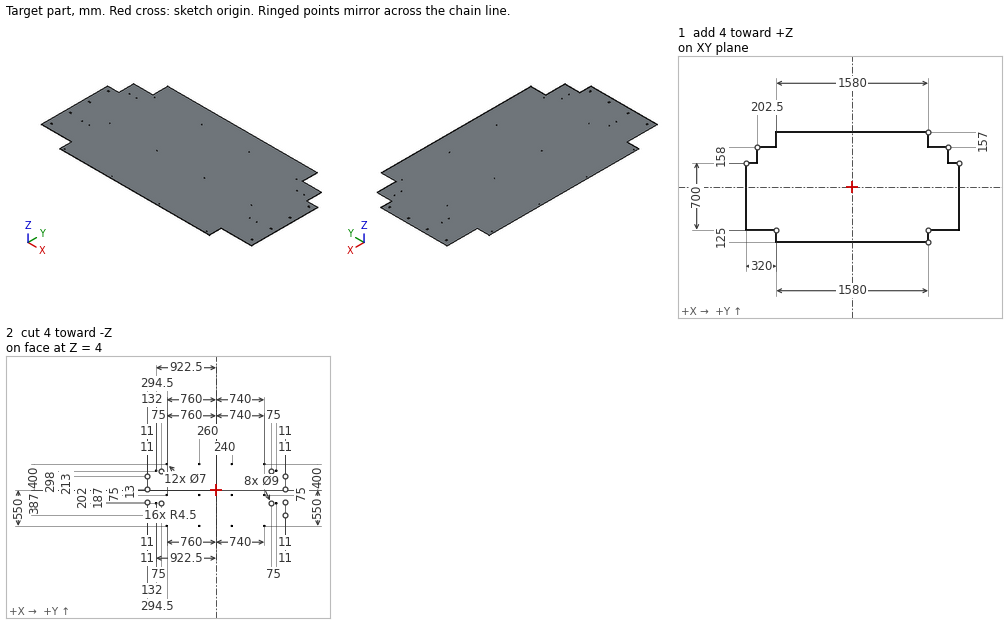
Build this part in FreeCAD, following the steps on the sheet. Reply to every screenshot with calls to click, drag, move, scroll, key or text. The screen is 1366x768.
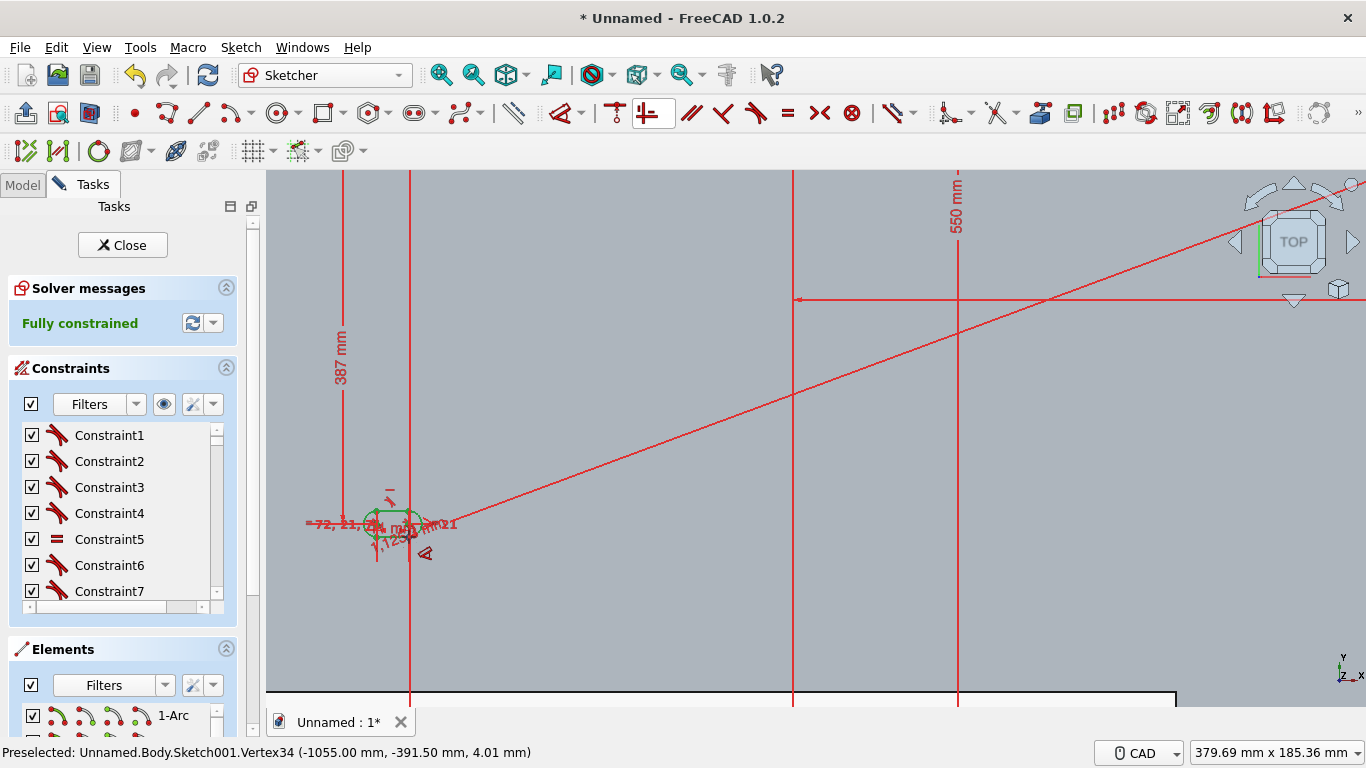
scroll(409, 540, down, 11)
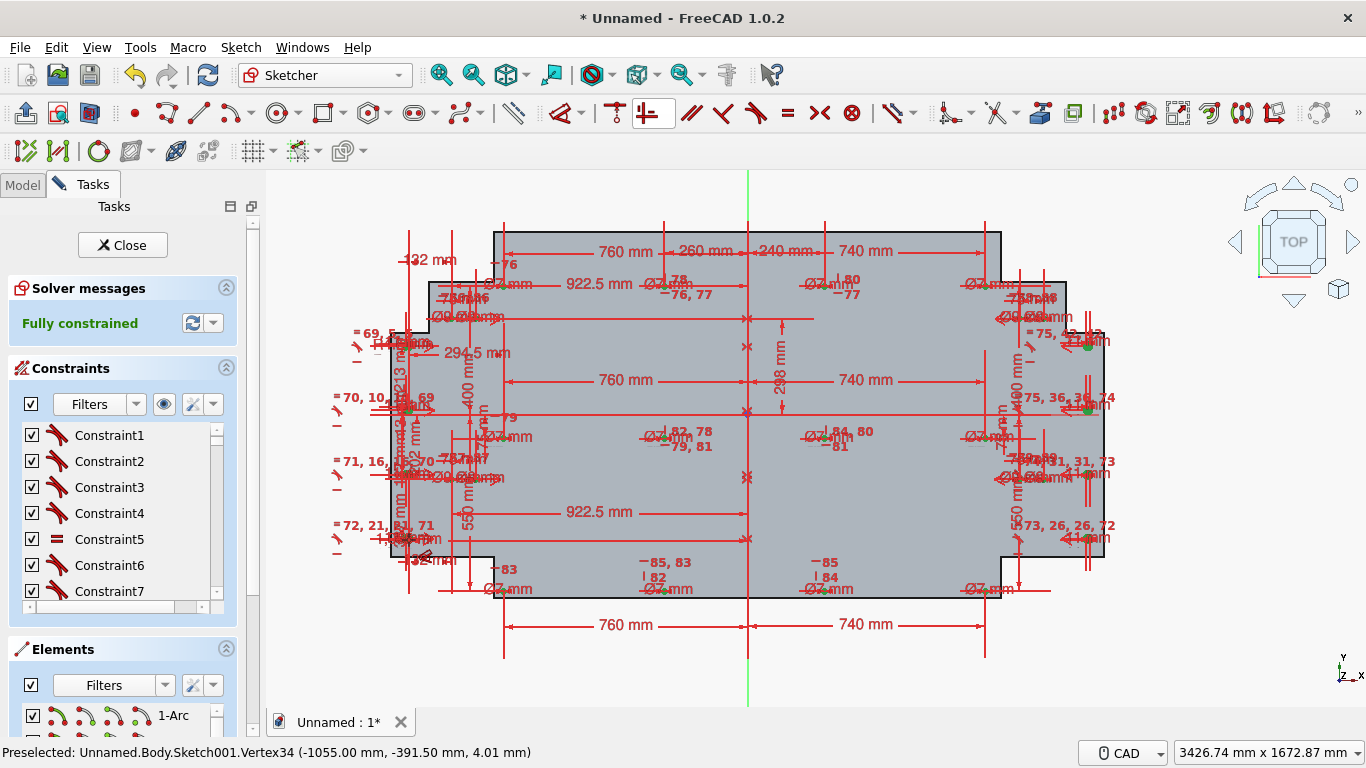
click(504, 591)
click(456, 625)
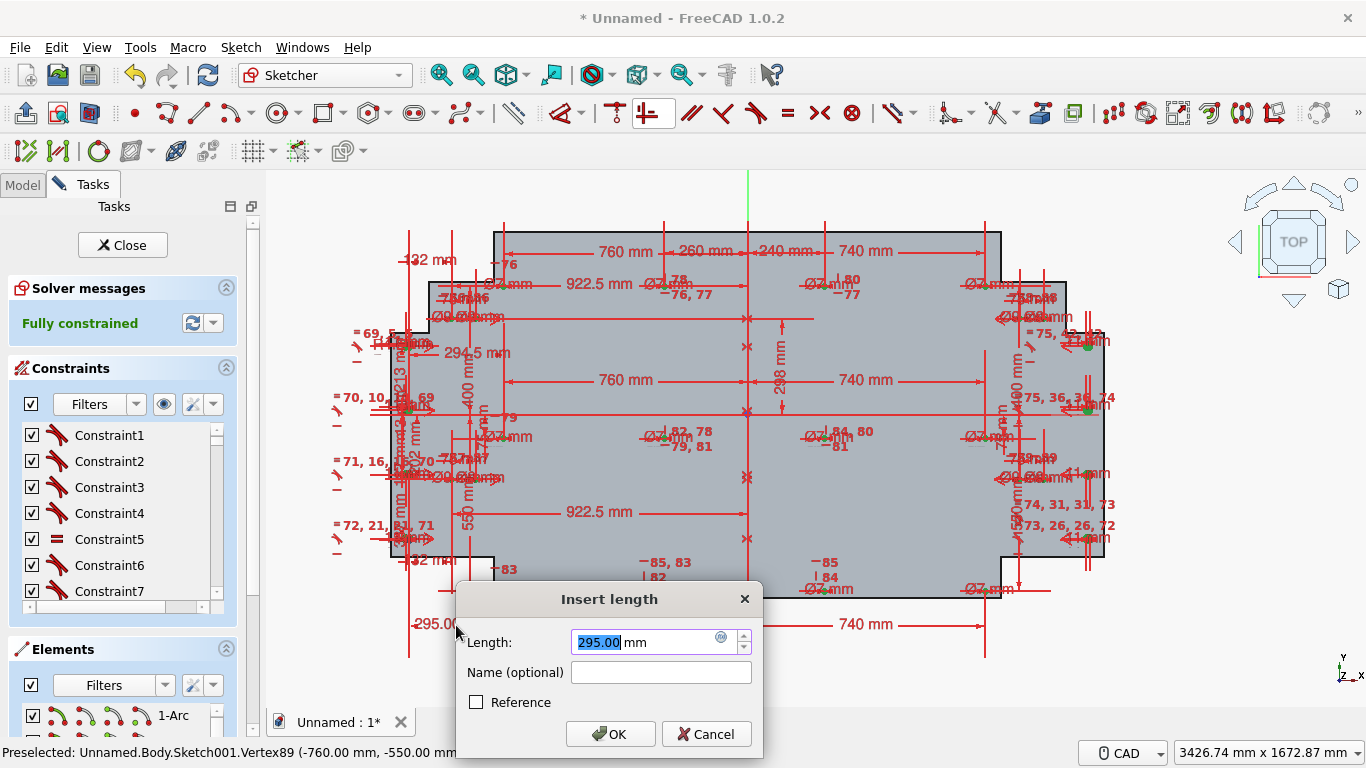
text(294.5)
key(Return)
key(Escape)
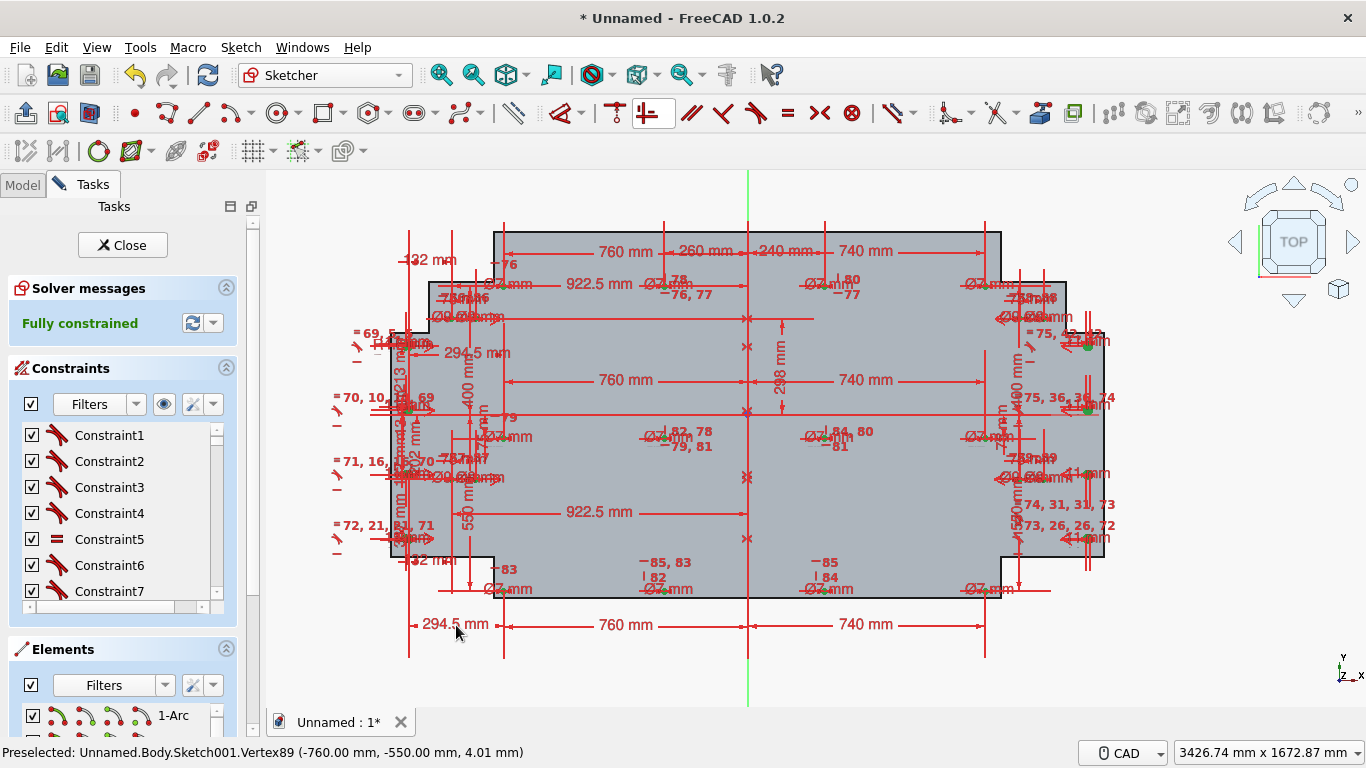
click(123, 245)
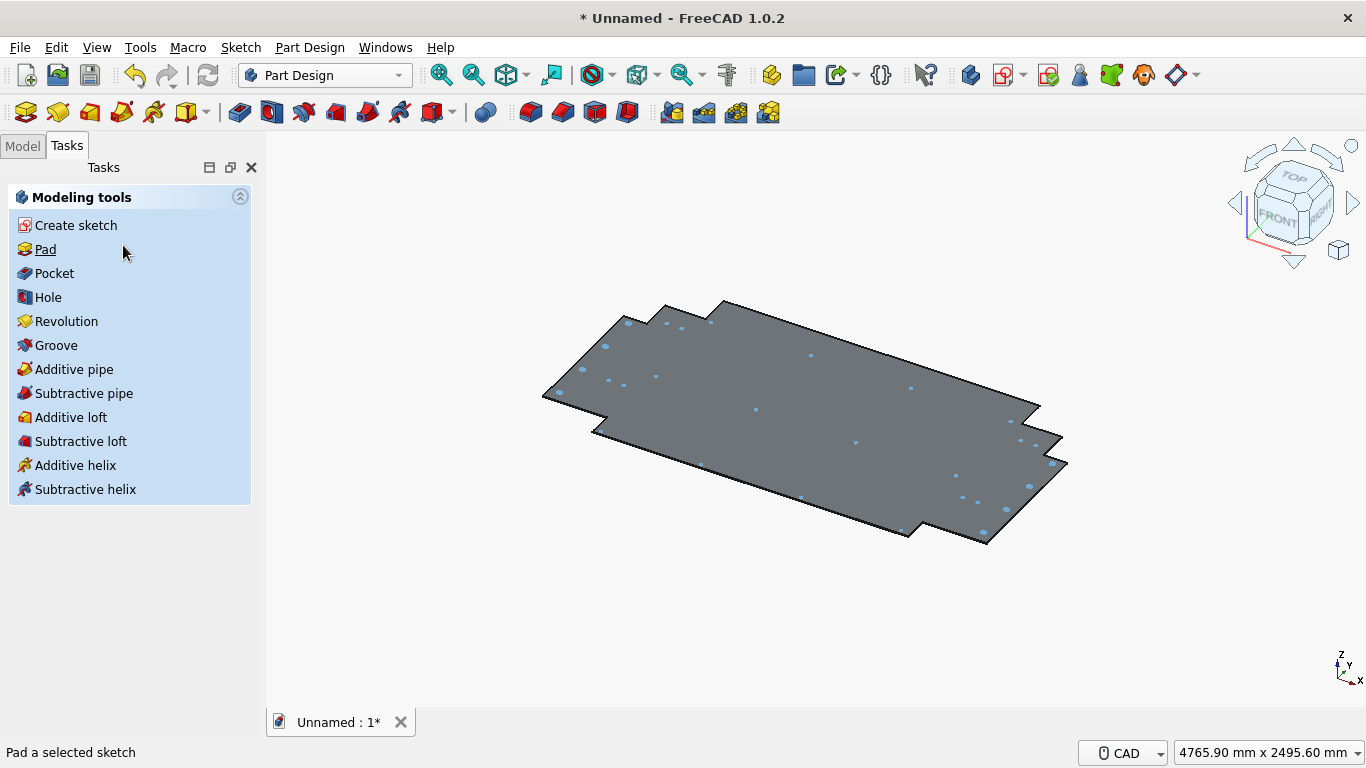
click(240, 112)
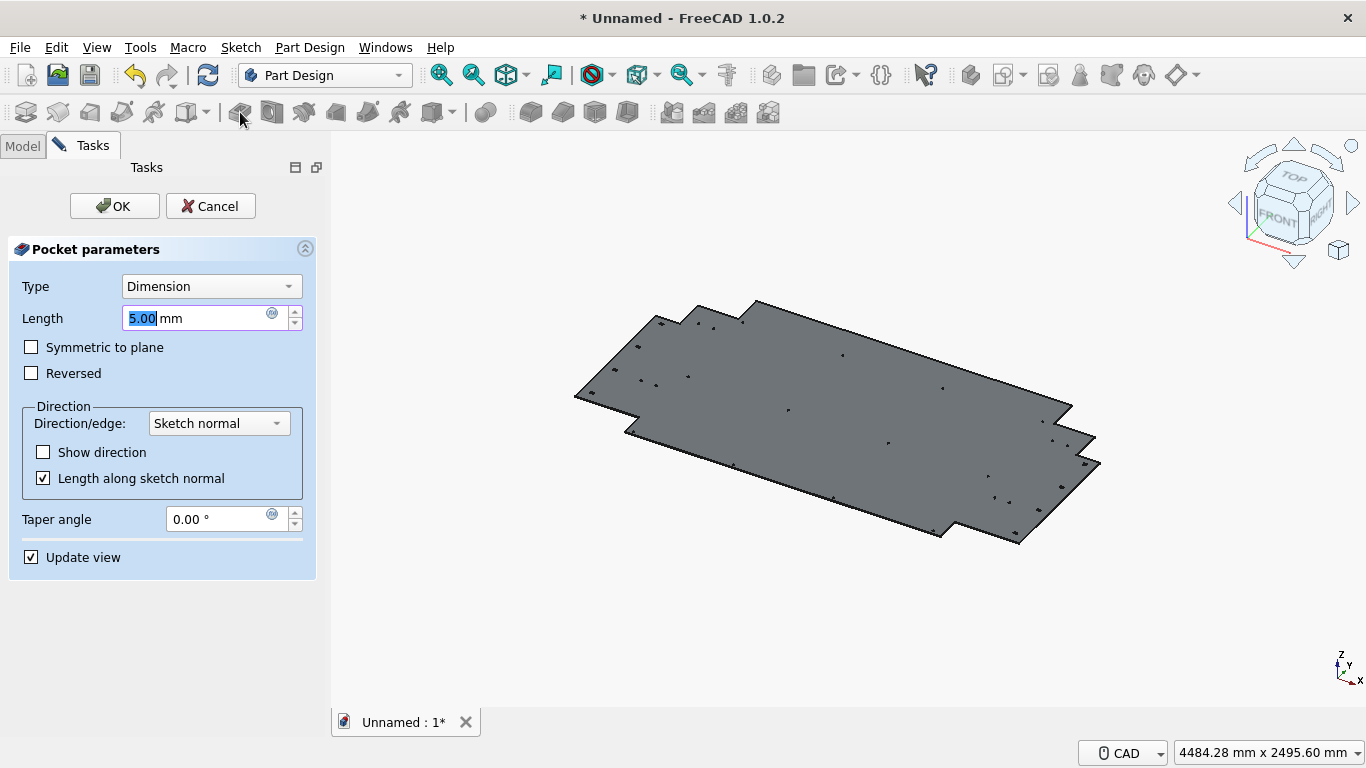
text(4)
key(Tab)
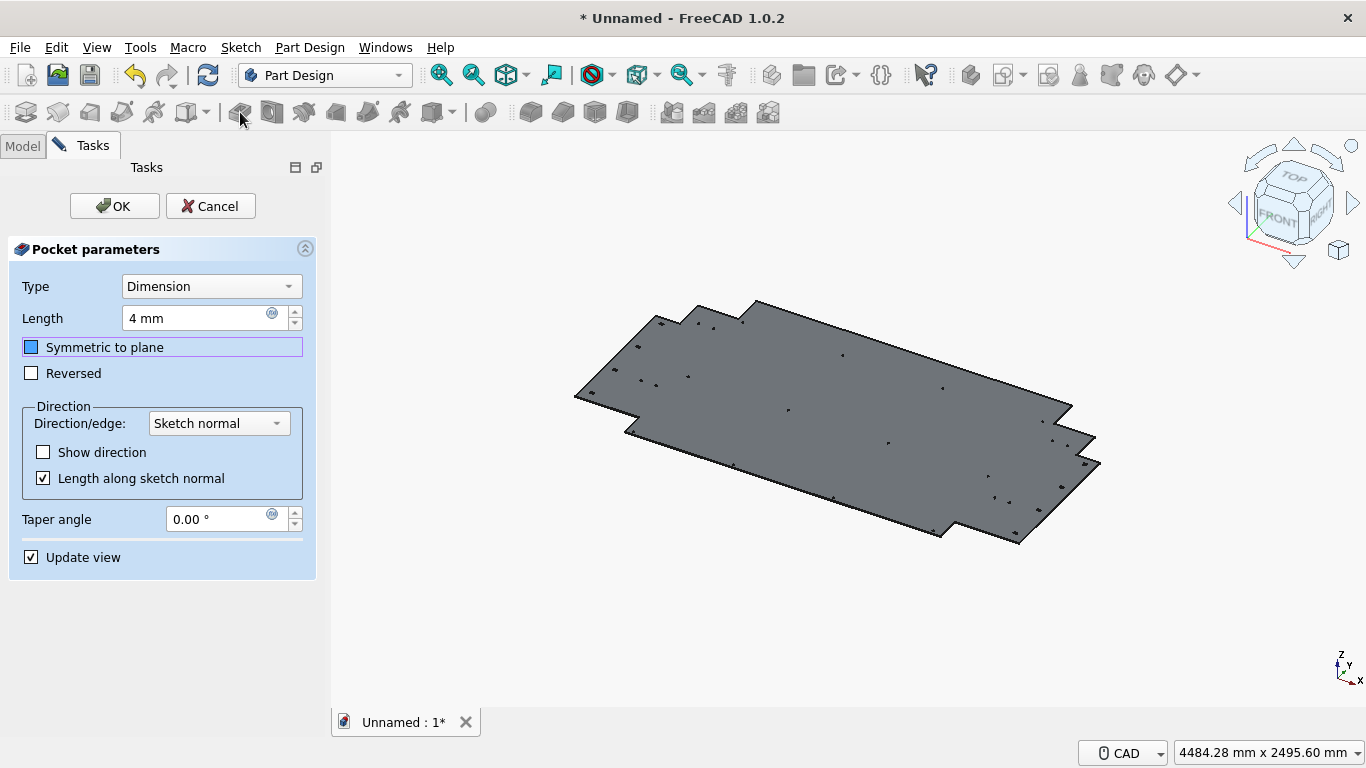
click(115, 206)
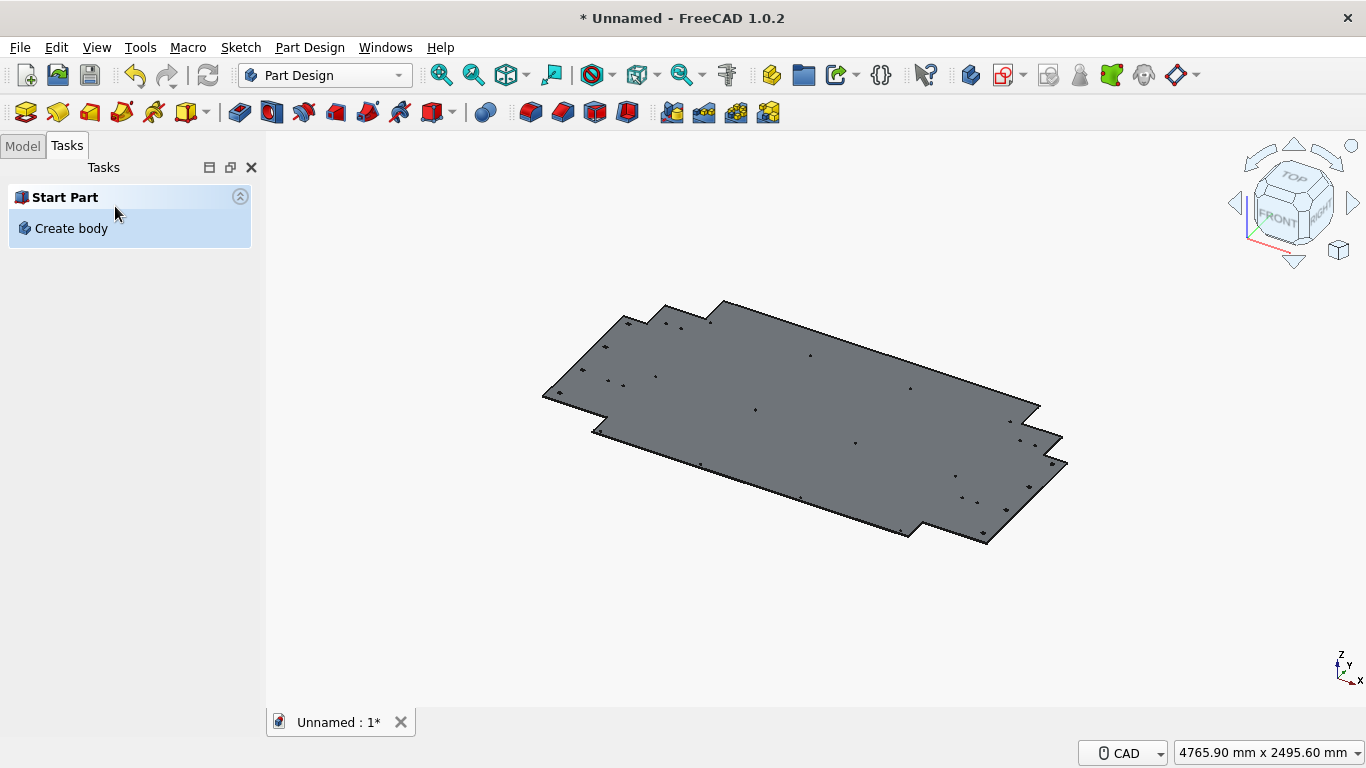
key(0)